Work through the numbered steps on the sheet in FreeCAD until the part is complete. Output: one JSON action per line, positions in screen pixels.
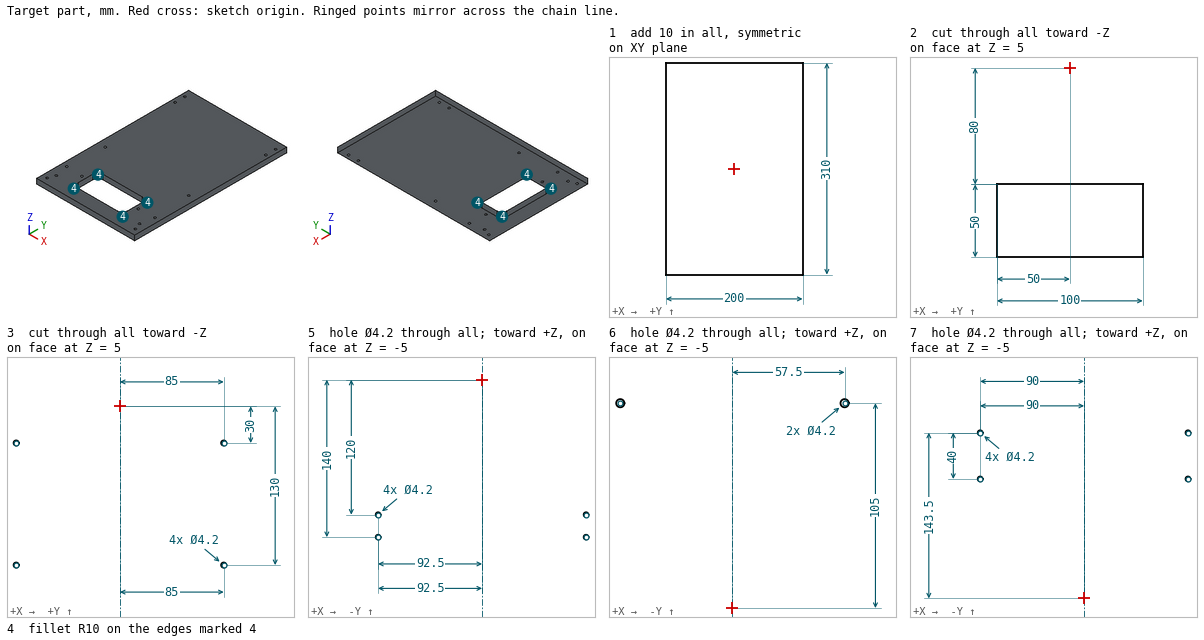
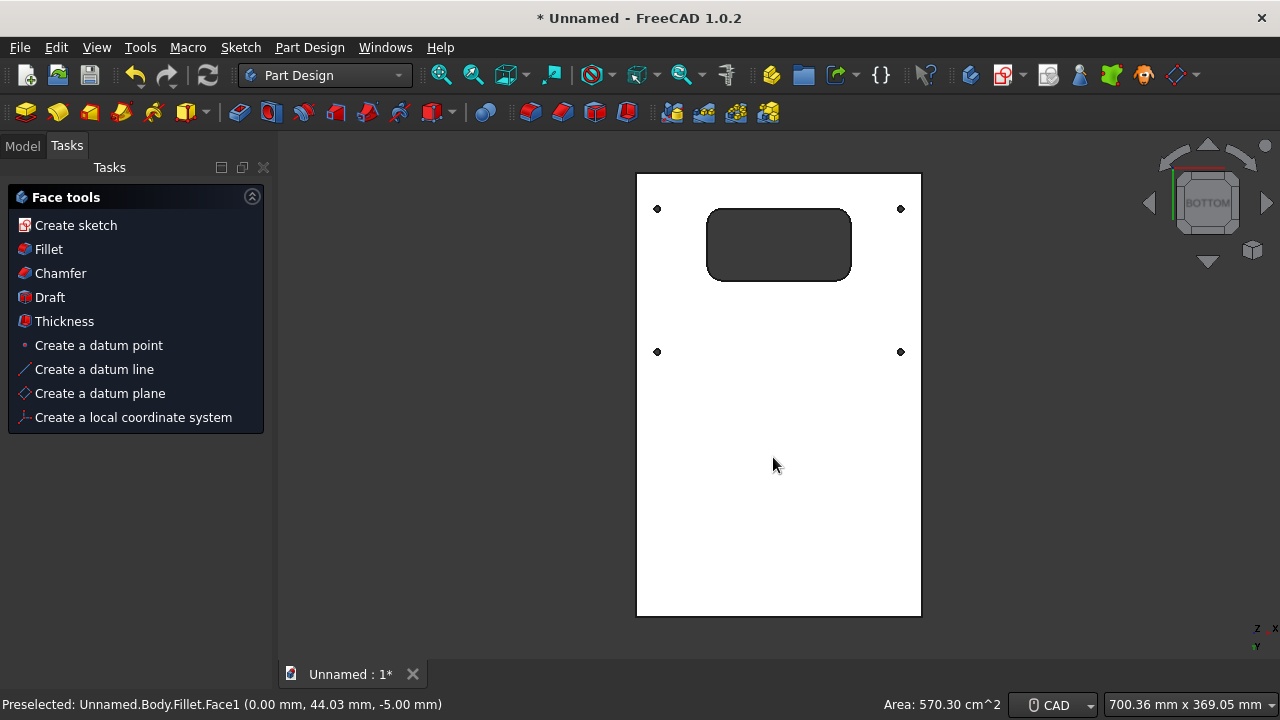
{"action": "left_click", "coordinate": [1004, 76]}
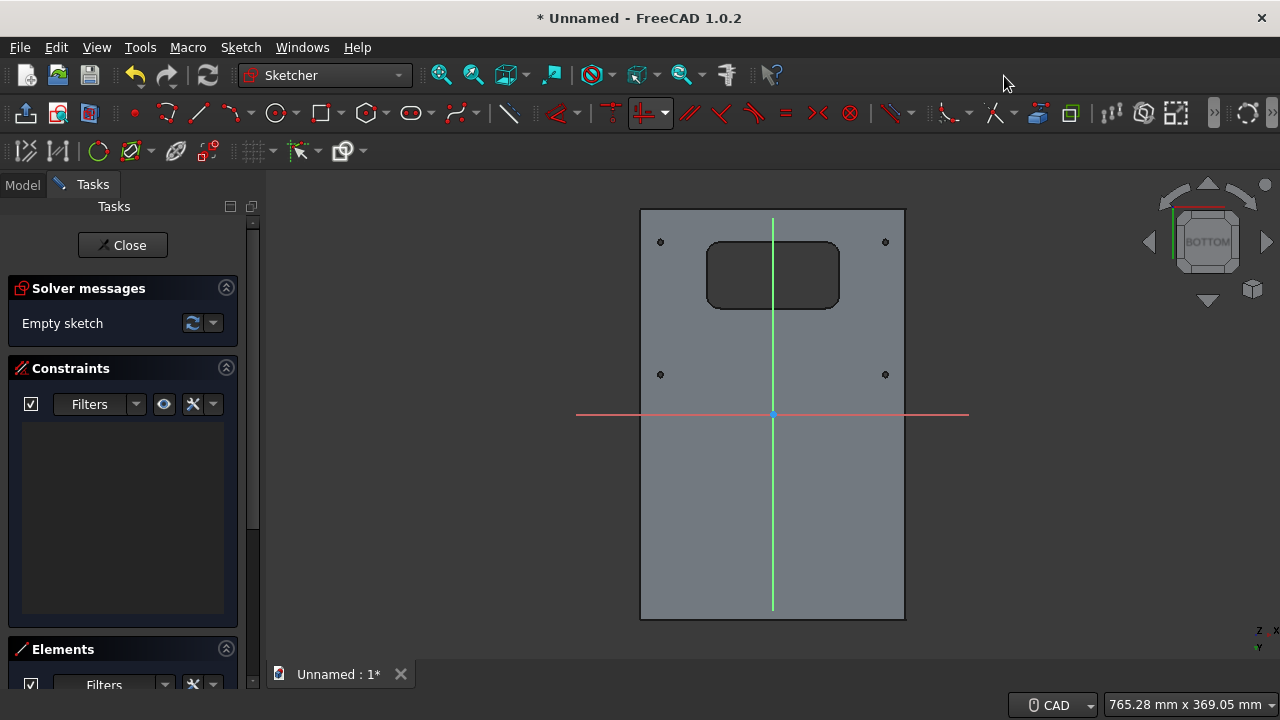
{"action": "scroll", "coordinate": [912, 631], "scroll_direction": "up", "scroll_amount": 2}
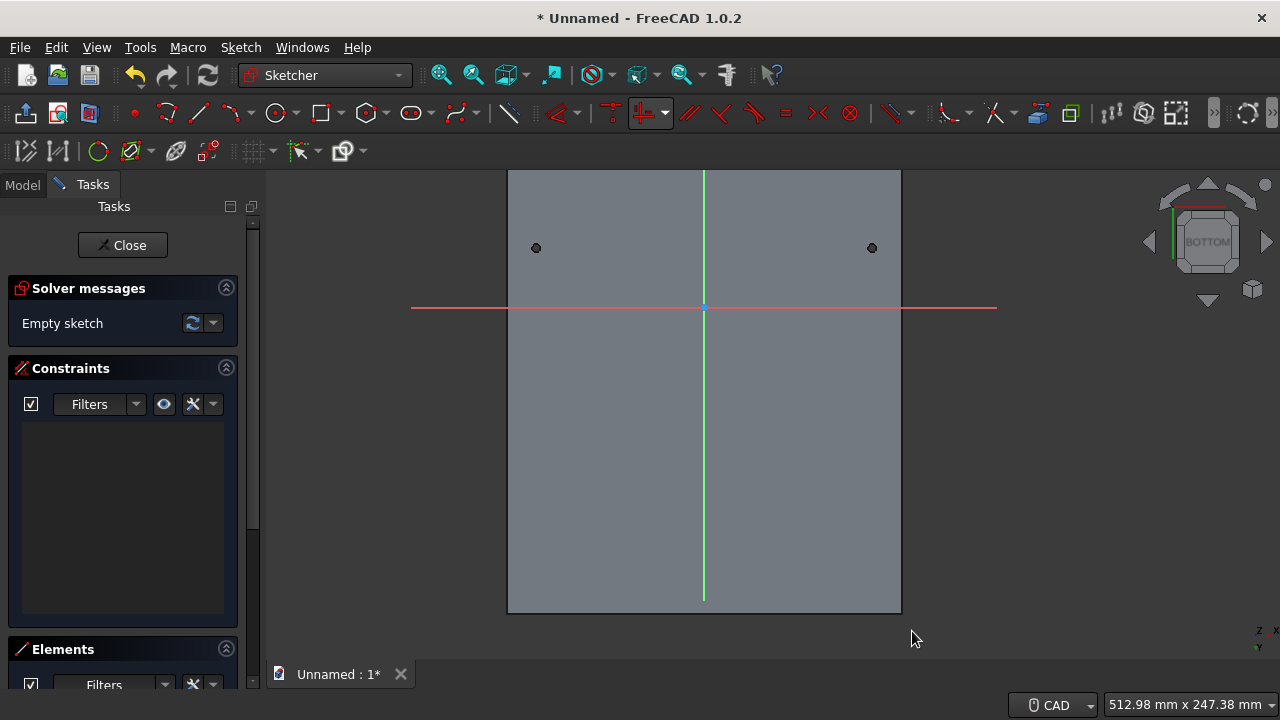
{"action": "left_click", "coordinate": [276, 114]}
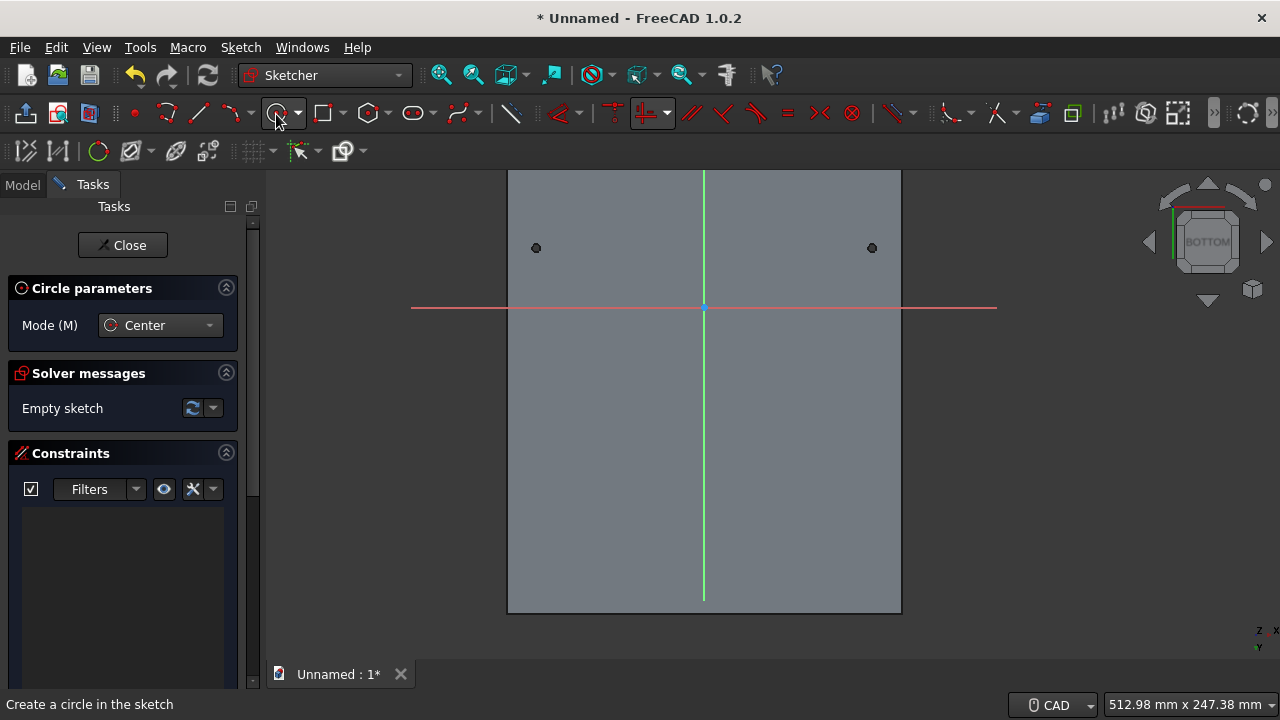
{"action": "scroll", "coordinate": [521, 545], "scroll_direction": "up", "scroll_amount": 9}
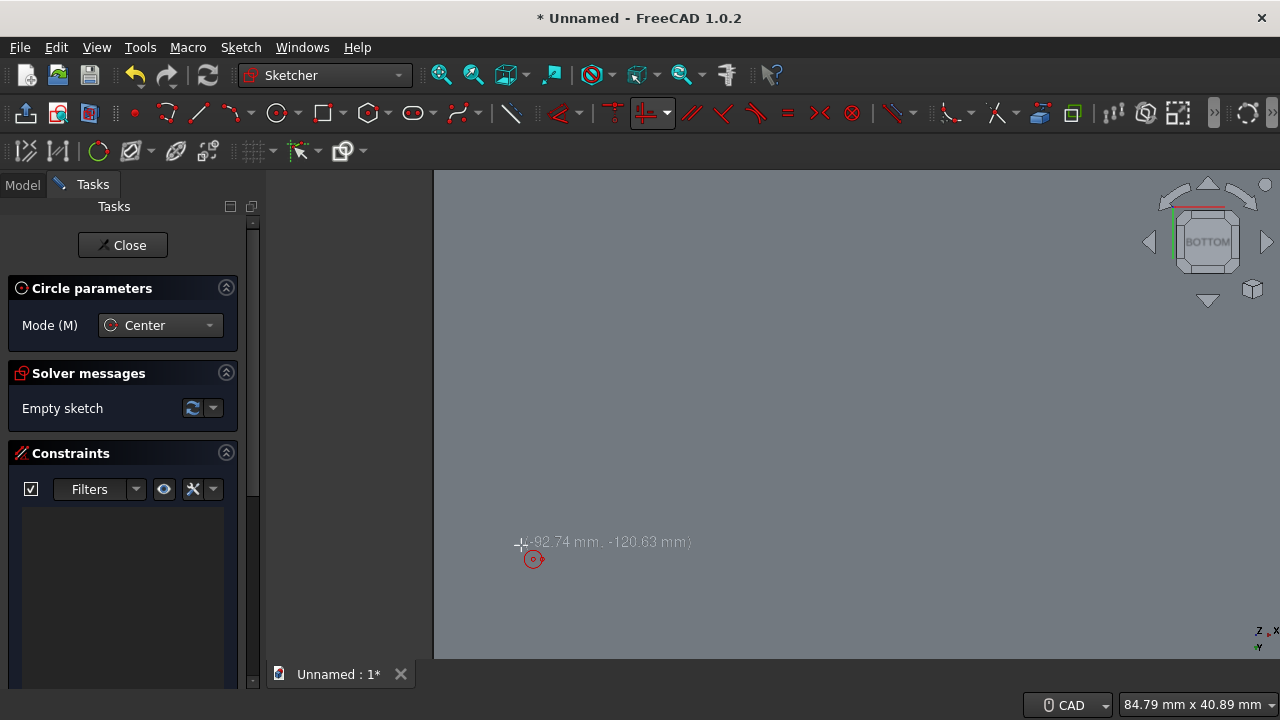
{"action": "scroll", "coordinate": [521, 506], "scroll_direction": "down", "scroll_amount": 9}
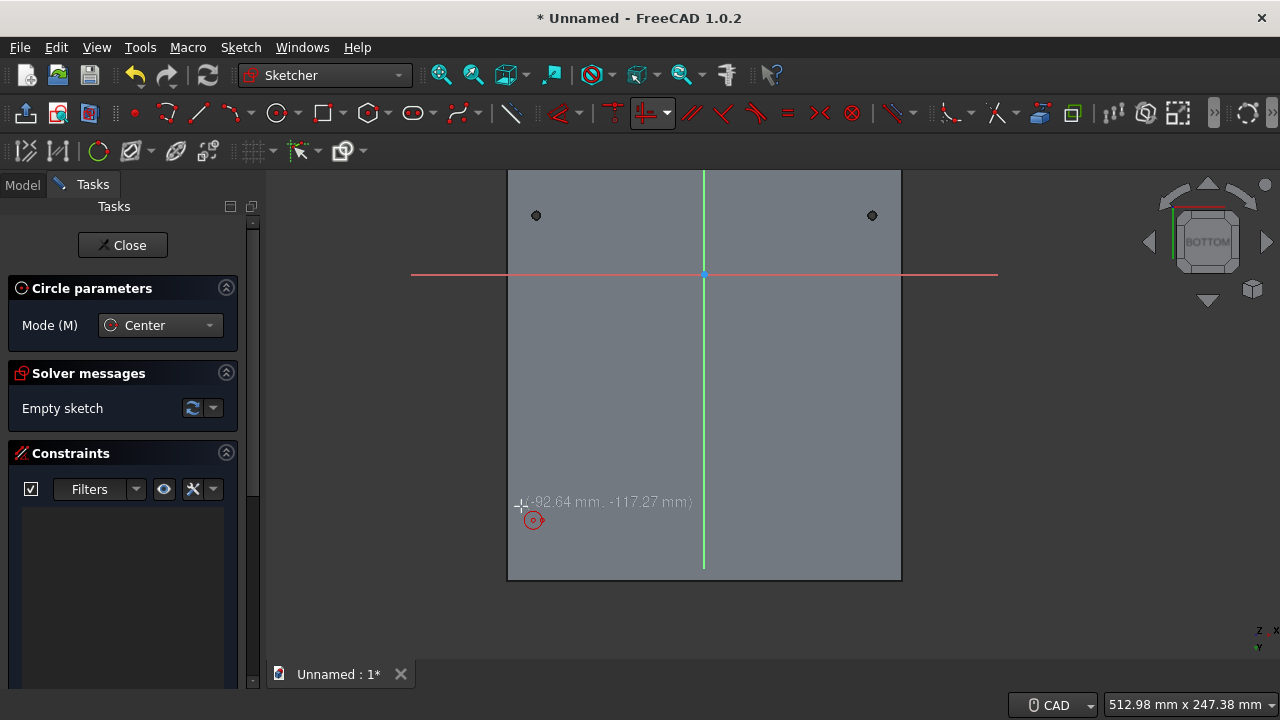
{"action": "left_click", "coordinate": [521, 512]}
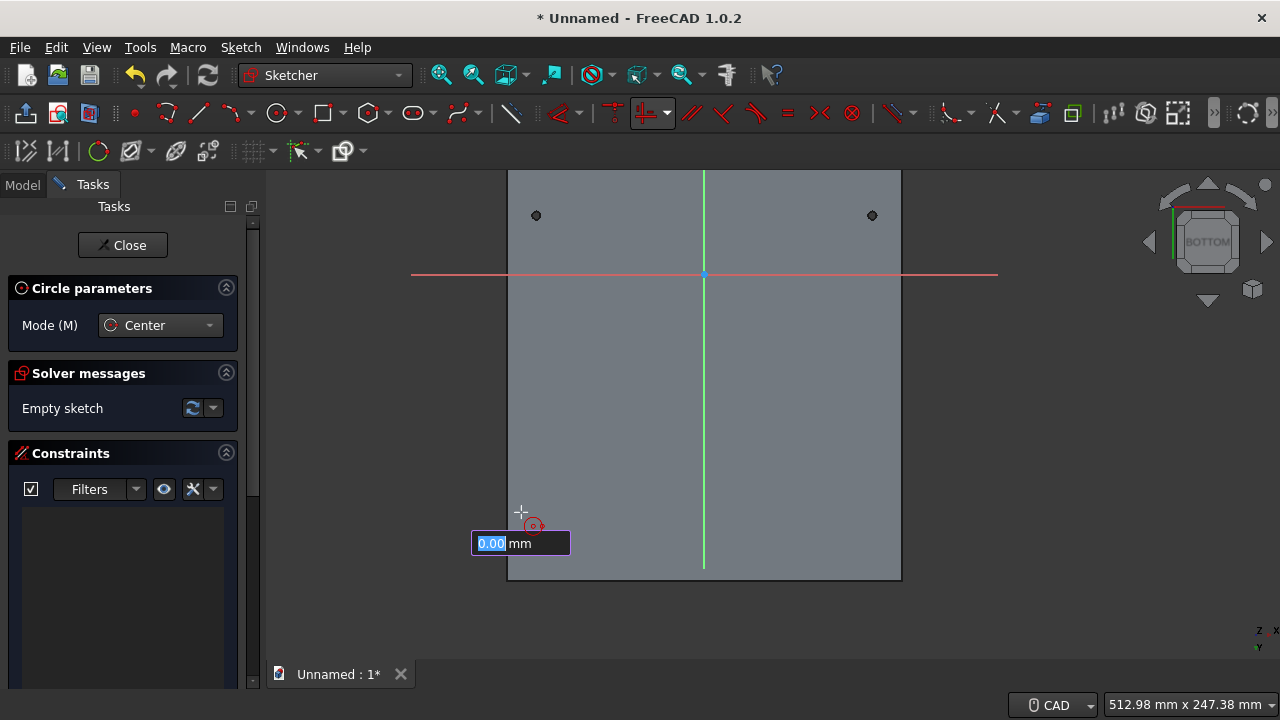
{"action": "scroll", "coordinate": [524, 509], "scroll_direction": "up", "scroll_amount": 7}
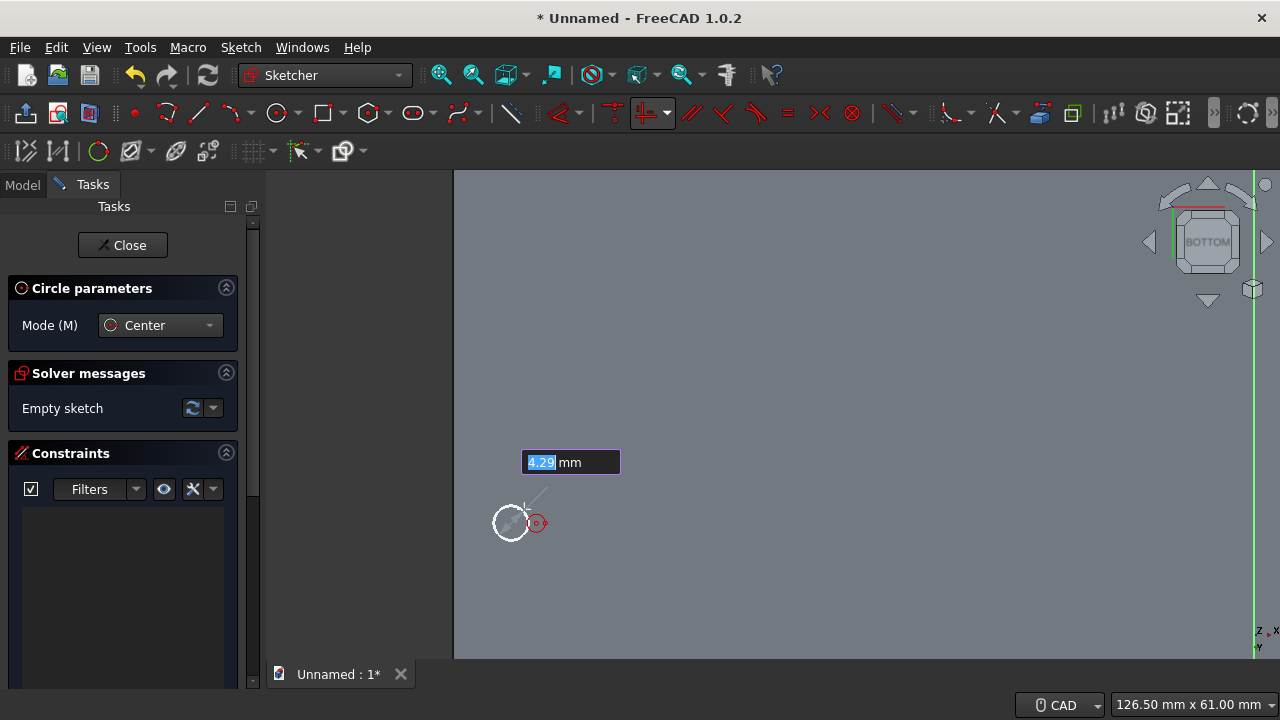
{"action": "left_click", "coordinate": [525, 508]}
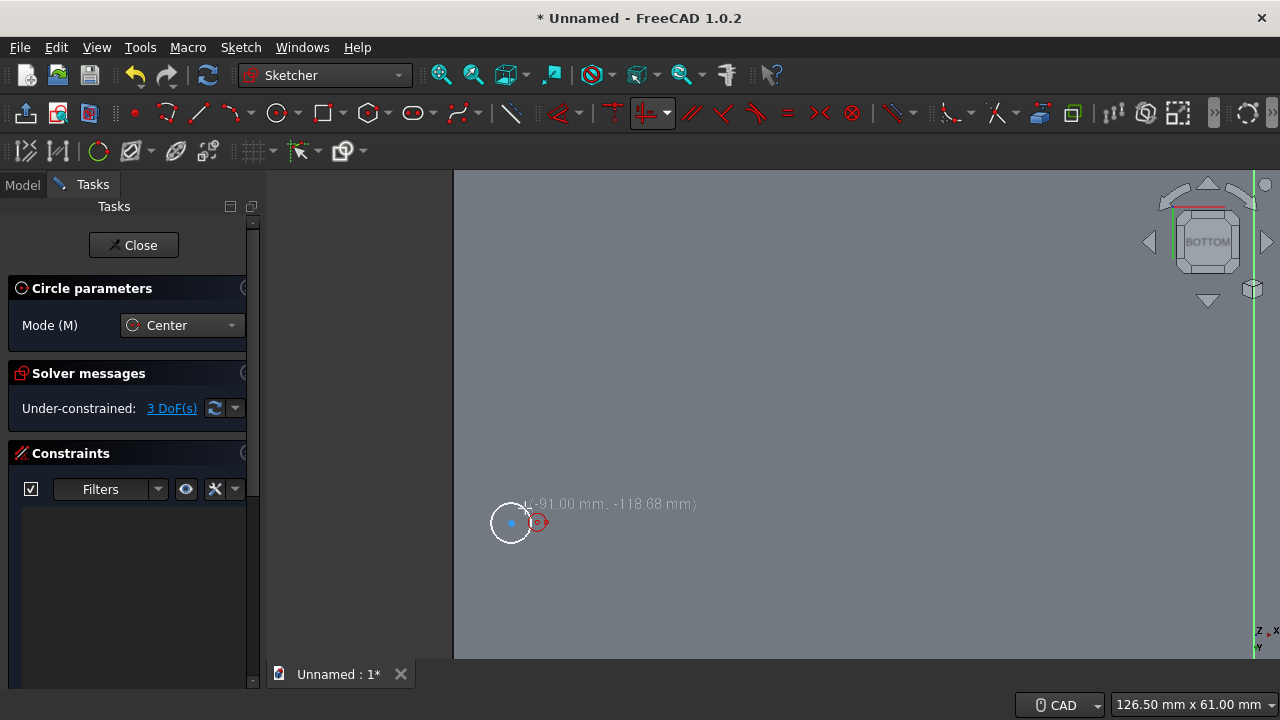
{"action": "scroll", "coordinate": [524, 509], "scroll_direction": "down", "scroll_amount": 7}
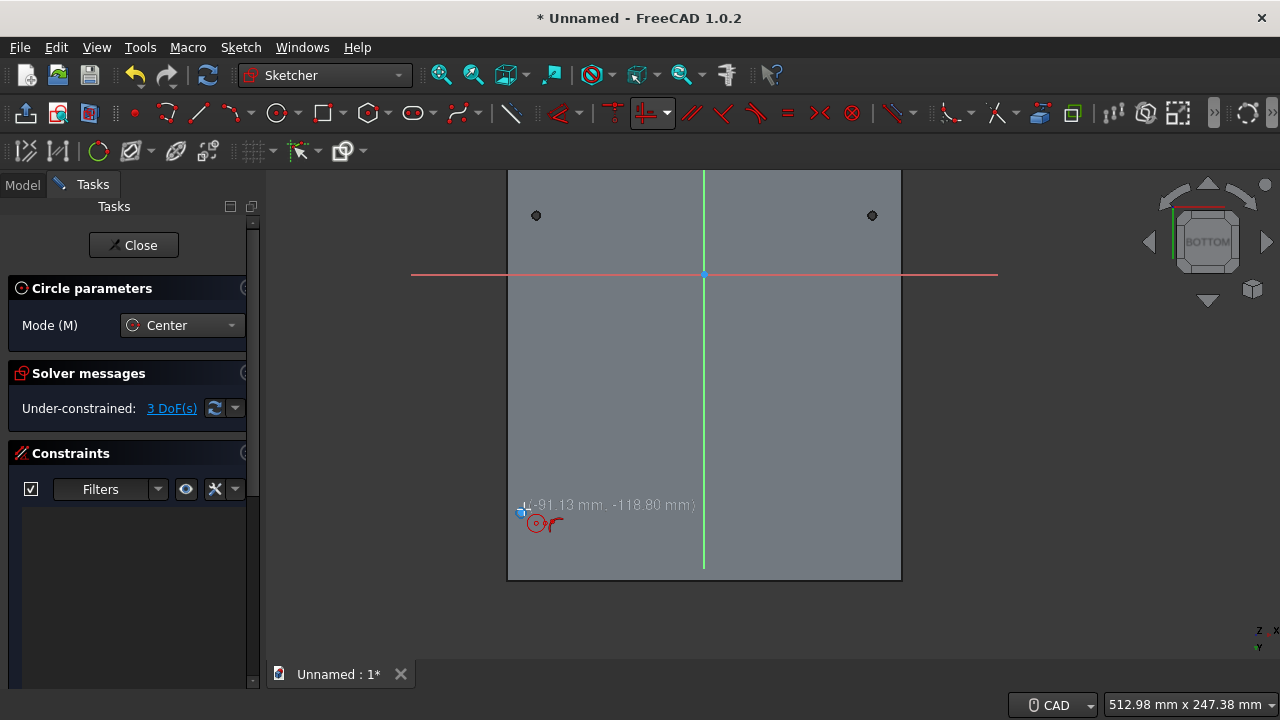
{"action": "scroll", "coordinate": [521, 552], "scroll_direction": "up", "scroll_amount": 9}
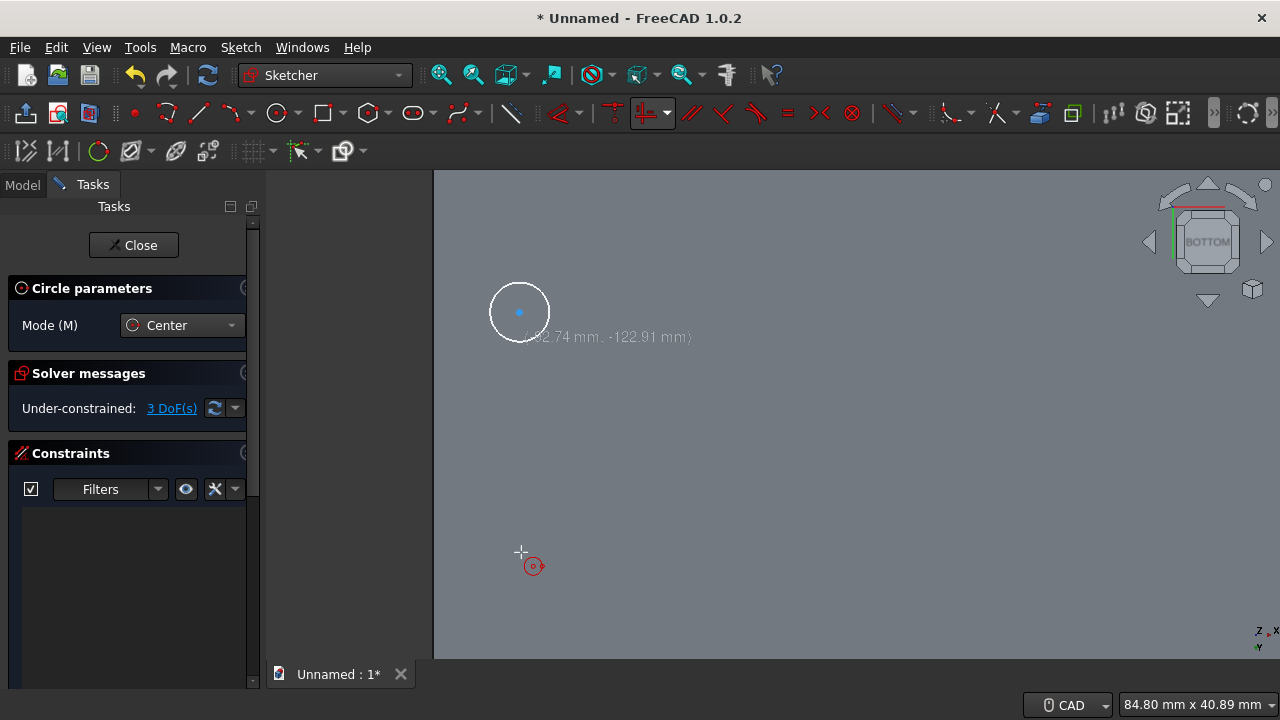
{"action": "scroll", "coordinate": [521, 552], "scroll_direction": "down", "scroll_amount": 9}